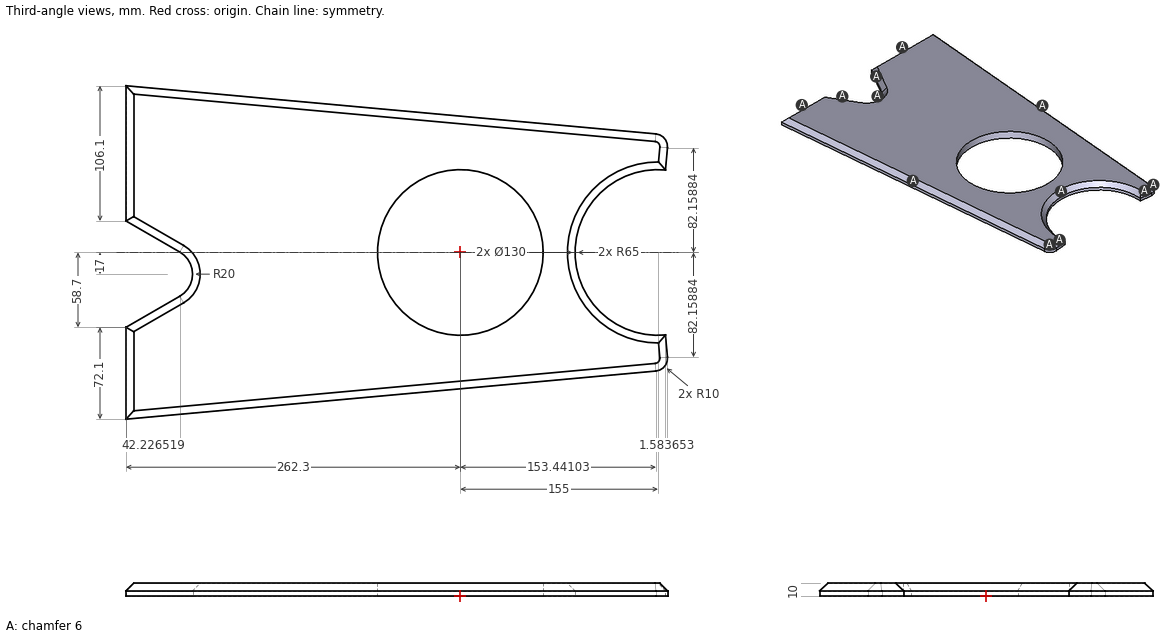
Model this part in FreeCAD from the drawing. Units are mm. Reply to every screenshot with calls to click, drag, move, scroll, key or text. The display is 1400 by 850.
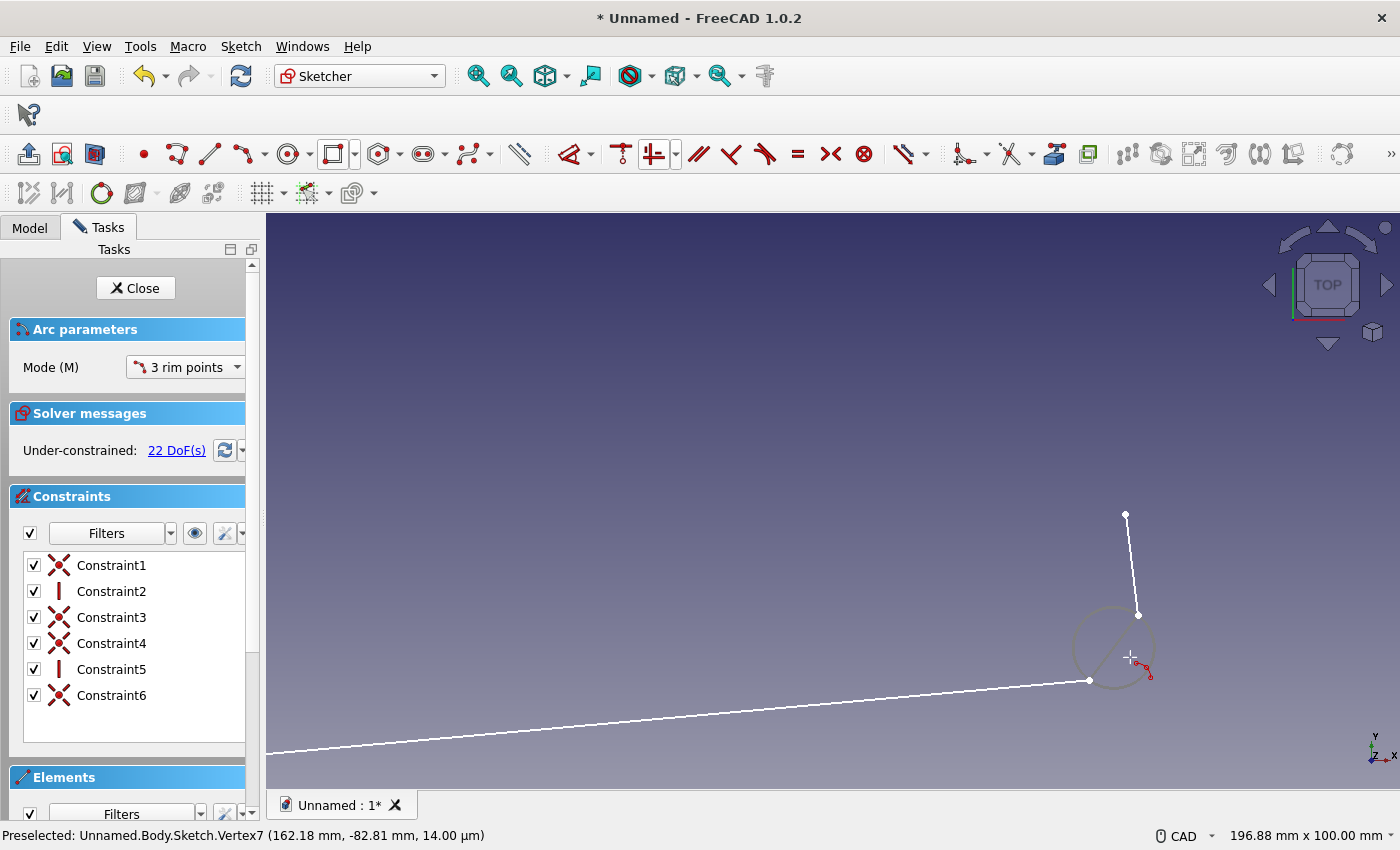
click(1127, 654)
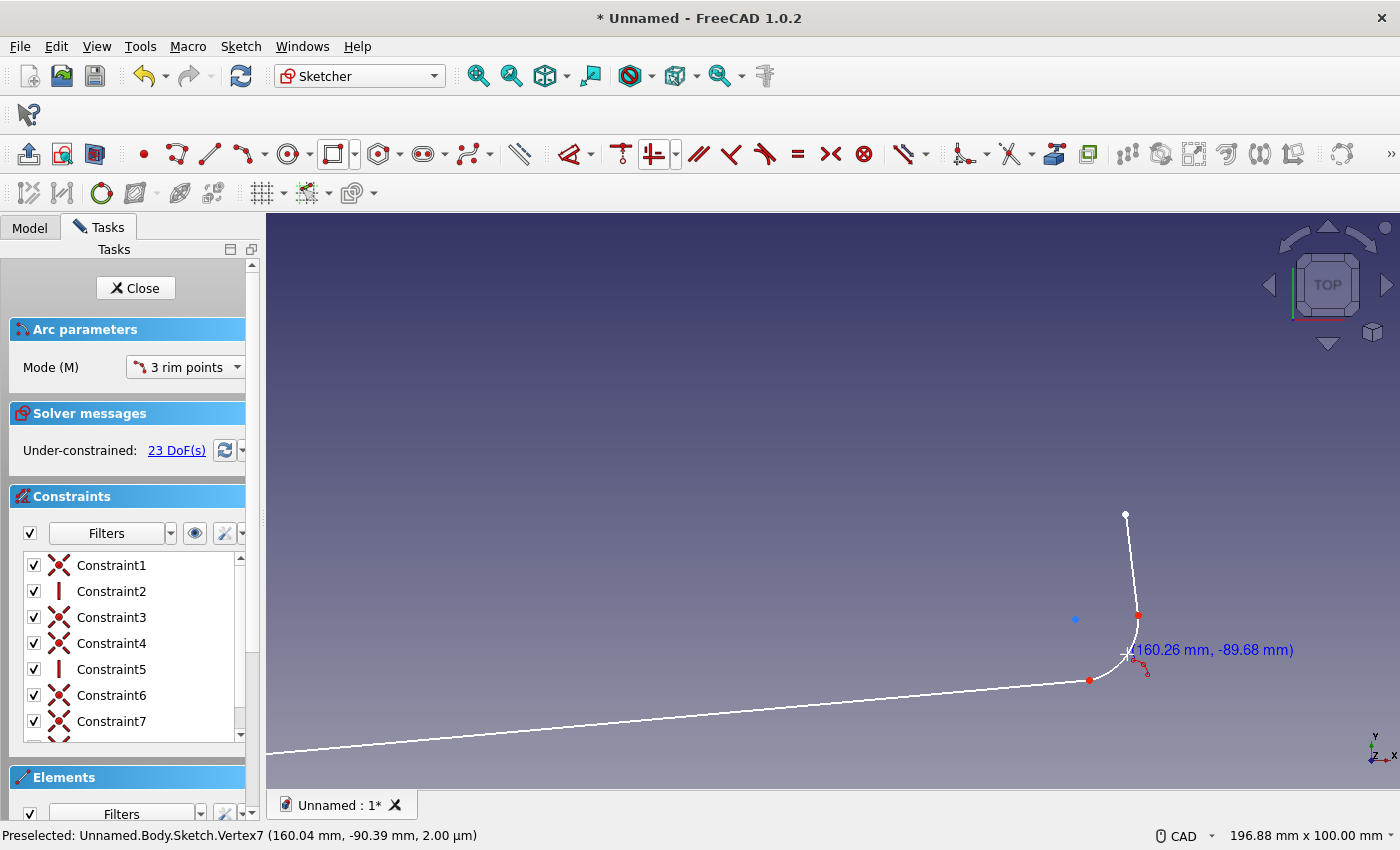
scroll(1042, 620, down, 7)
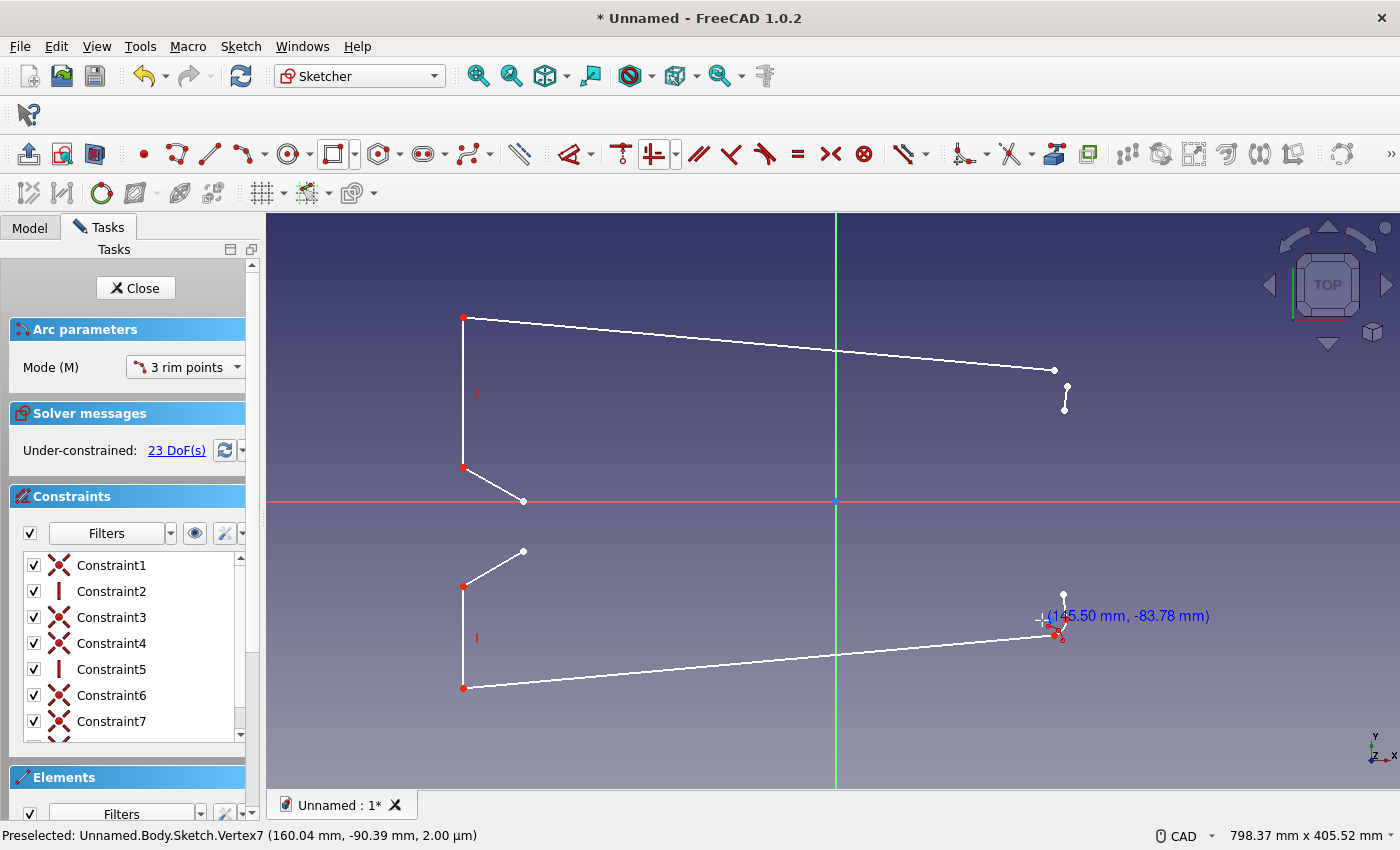
scroll(1064, 594, up, 2)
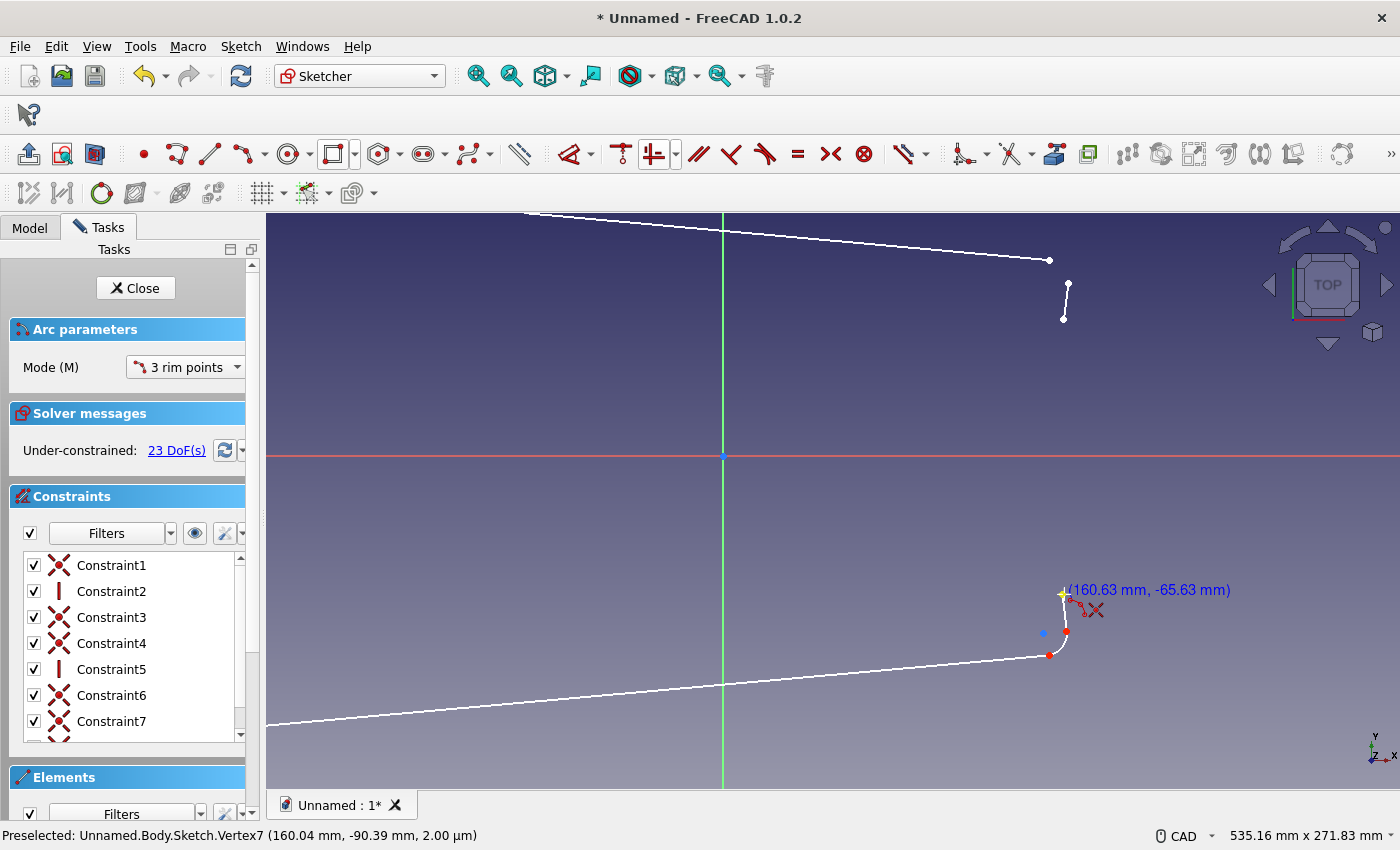
click(1062, 594)
click(1064, 320)
click(922, 411)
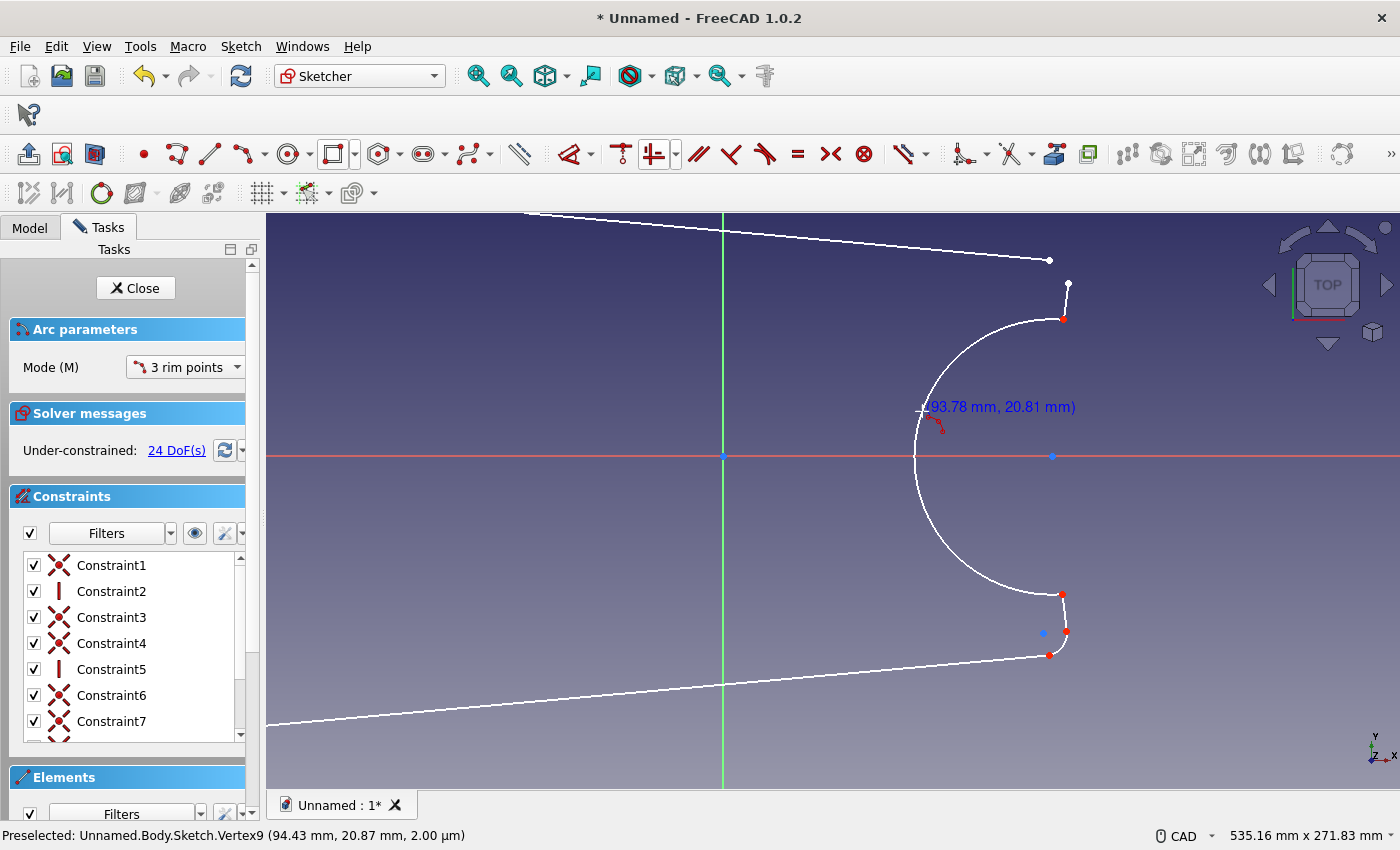
click(1068, 284)
click(1049, 260)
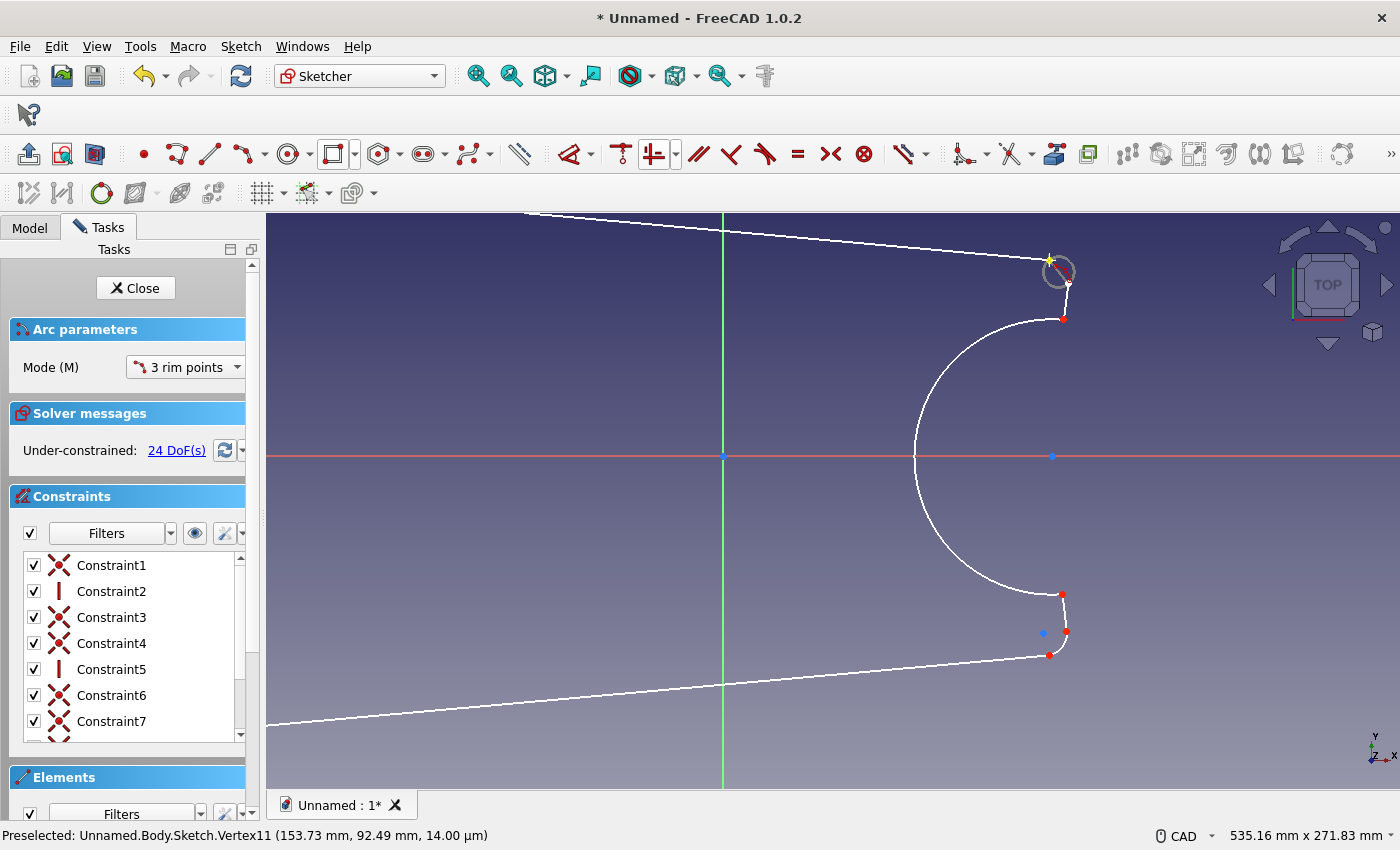
scroll(1063, 267, up, 5)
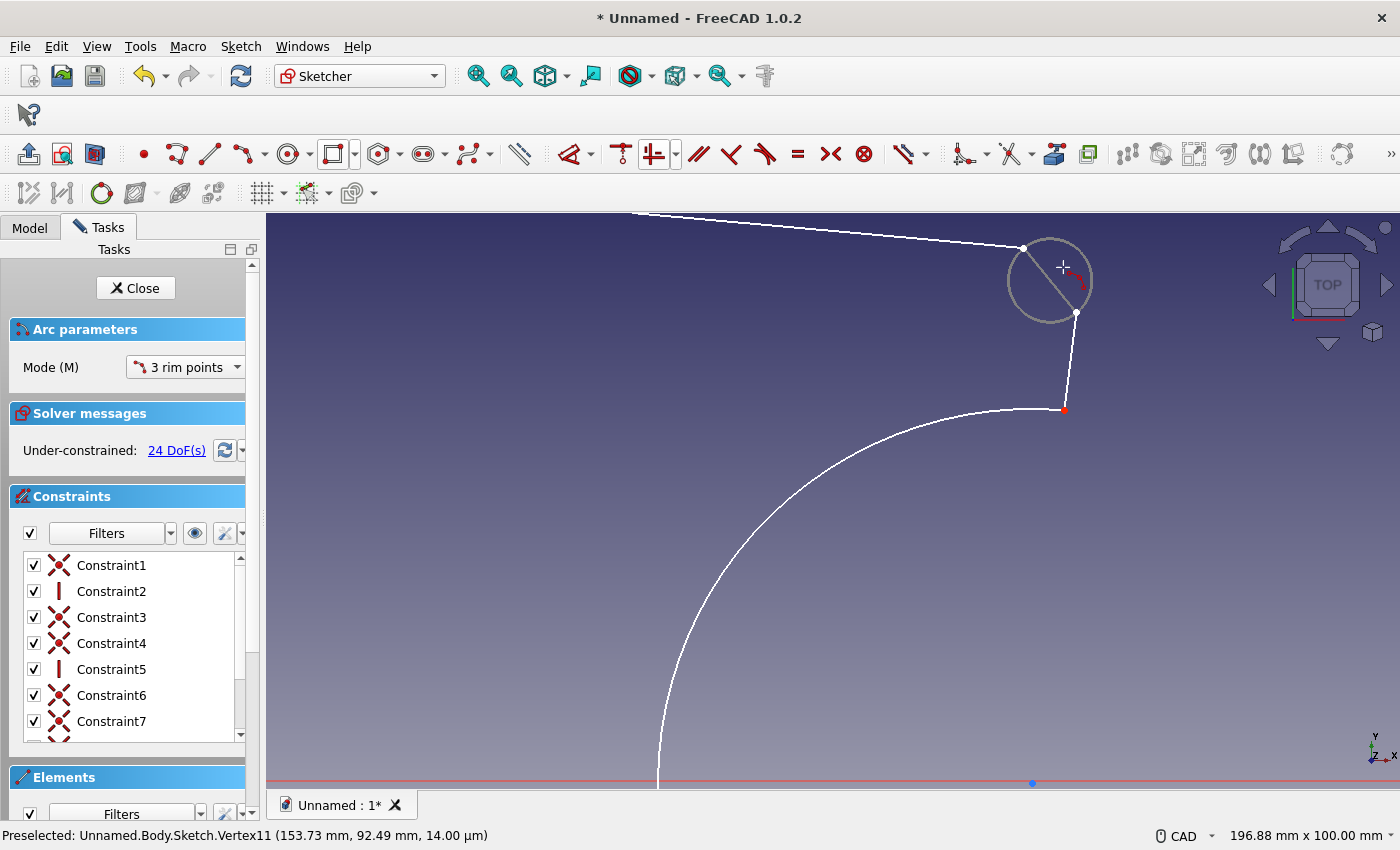
click(1061, 266)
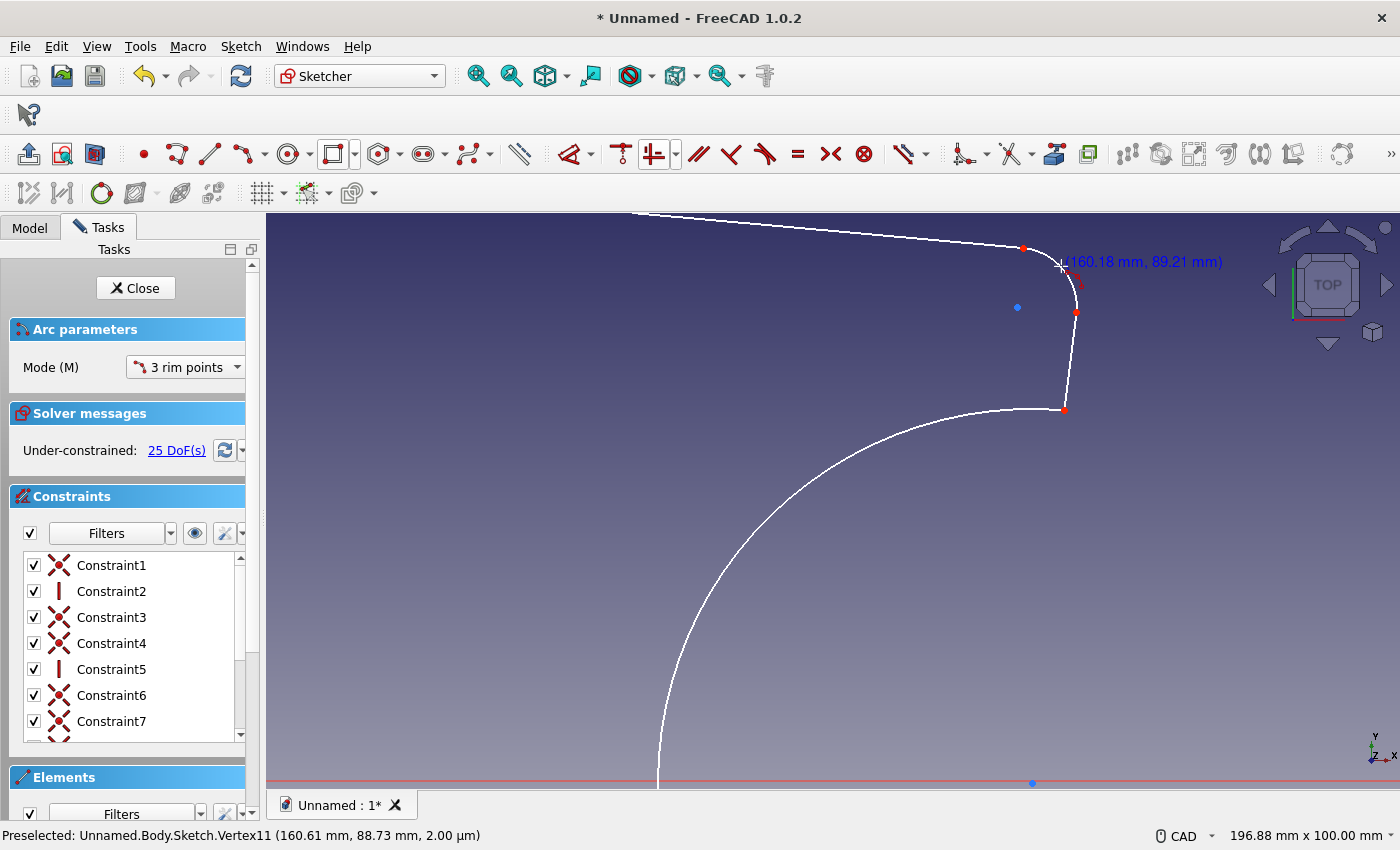
scroll(1064, 409, down, 7)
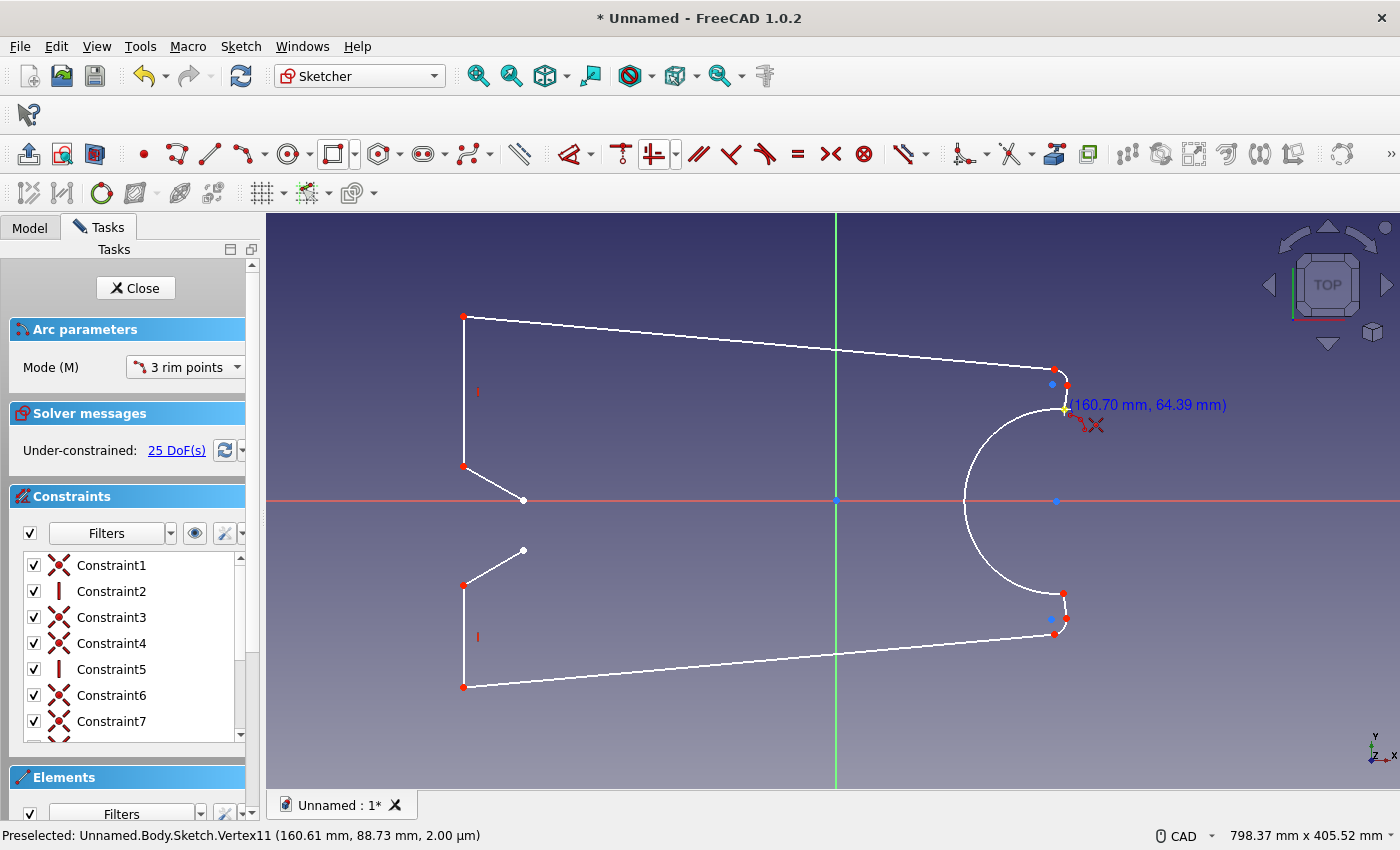
scroll(524, 501, up, 18)